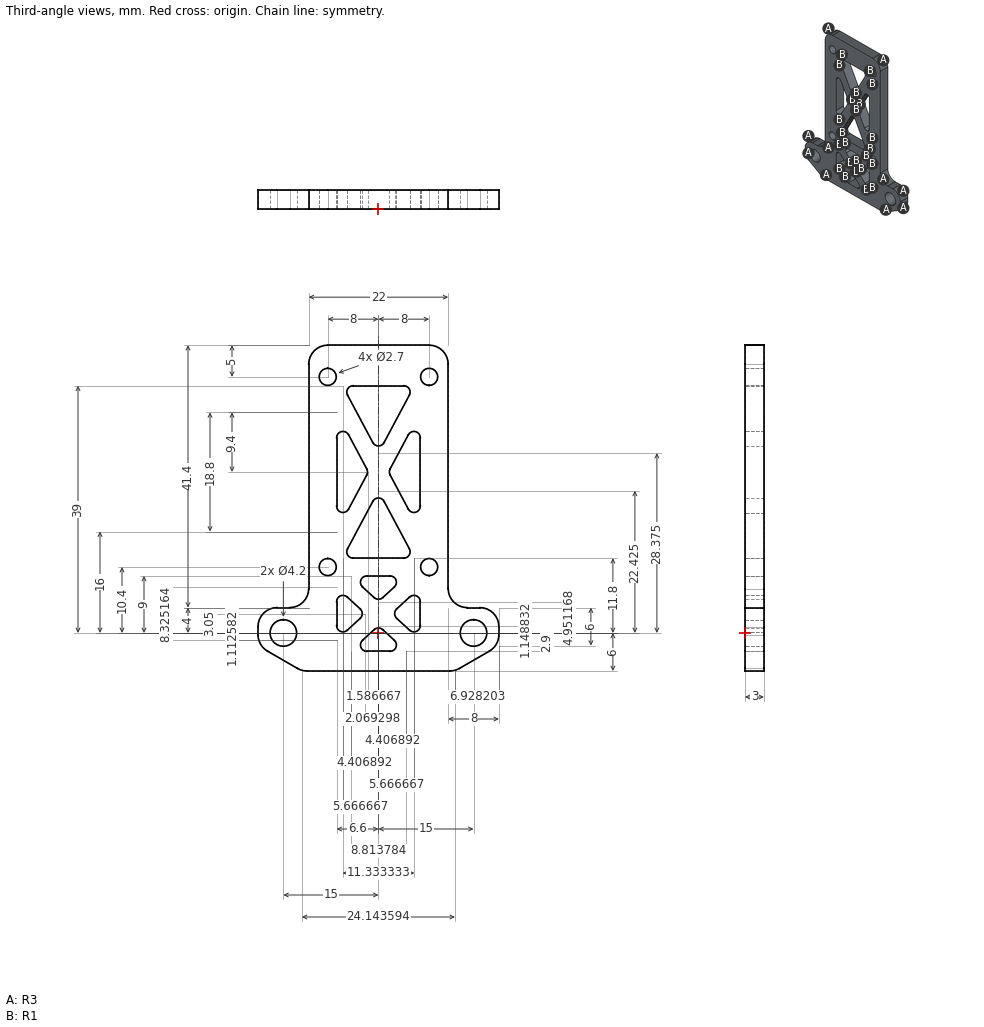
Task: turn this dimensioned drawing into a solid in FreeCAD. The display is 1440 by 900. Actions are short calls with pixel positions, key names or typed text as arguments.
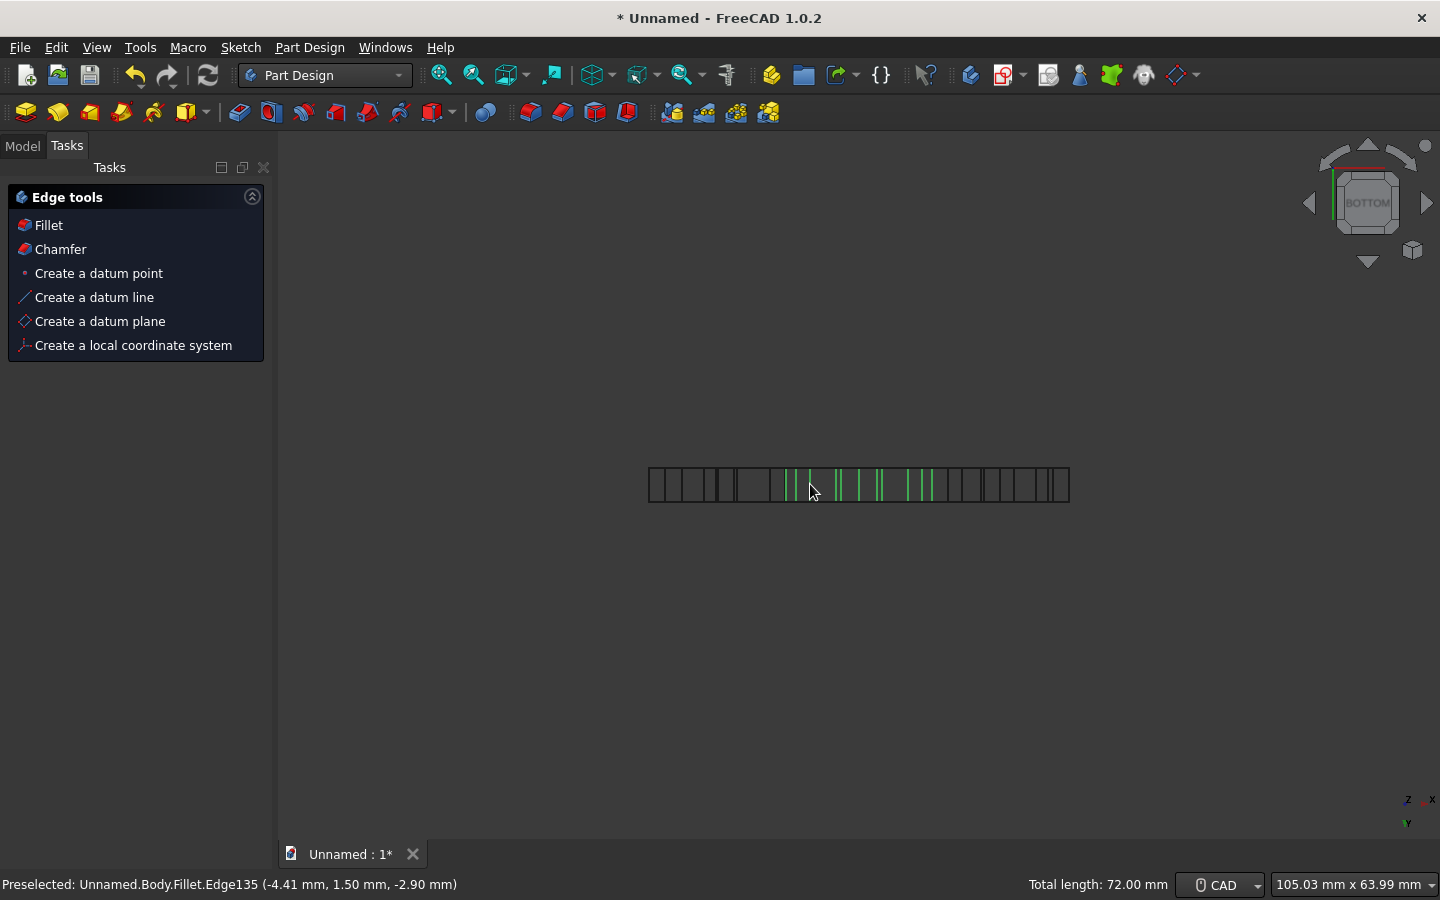
key(v)
key(1)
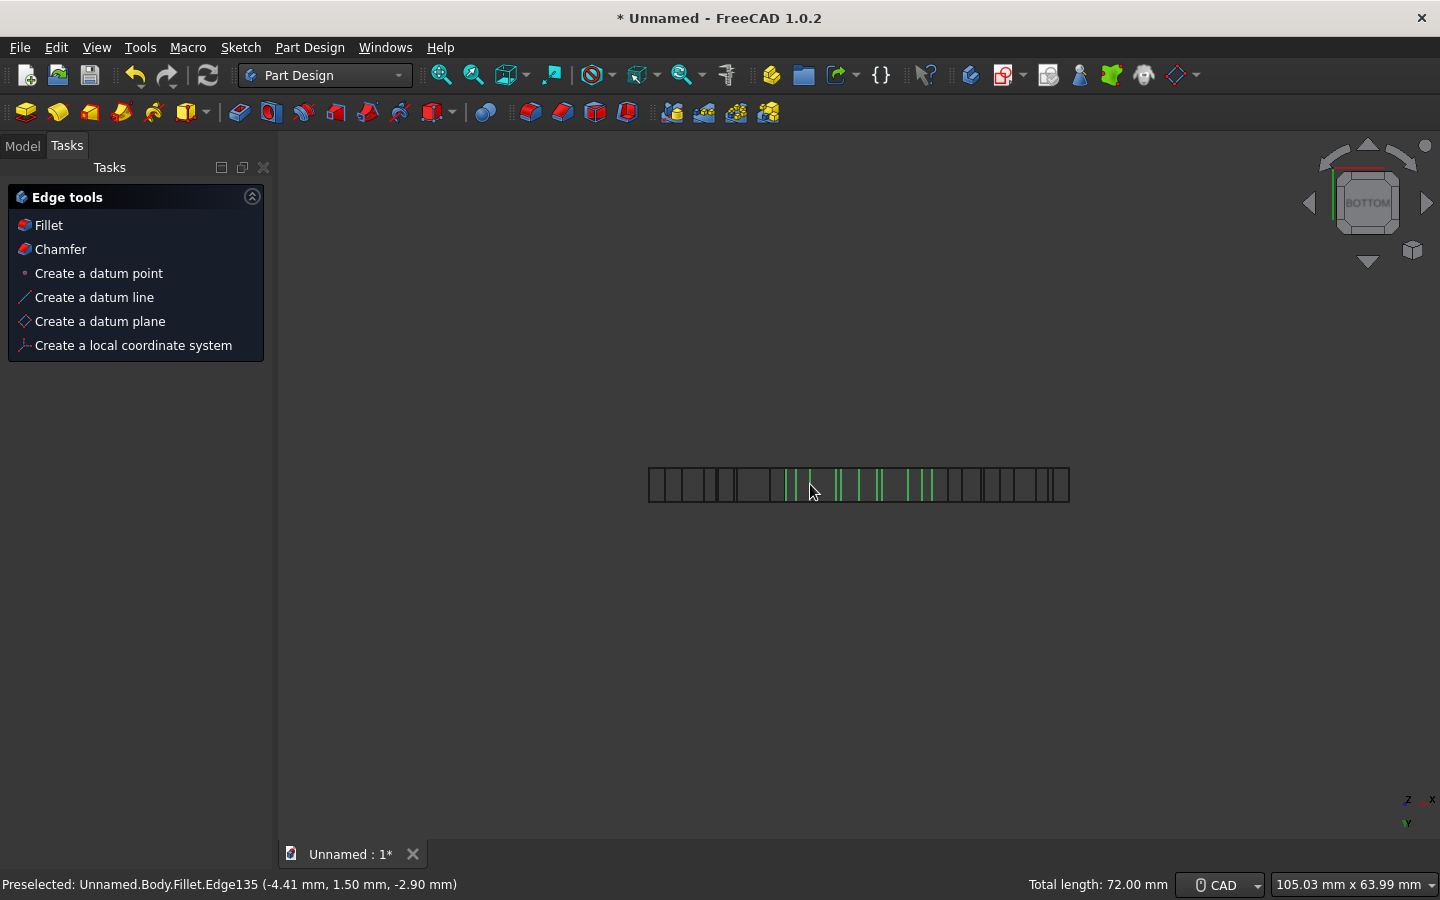
click(532, 112)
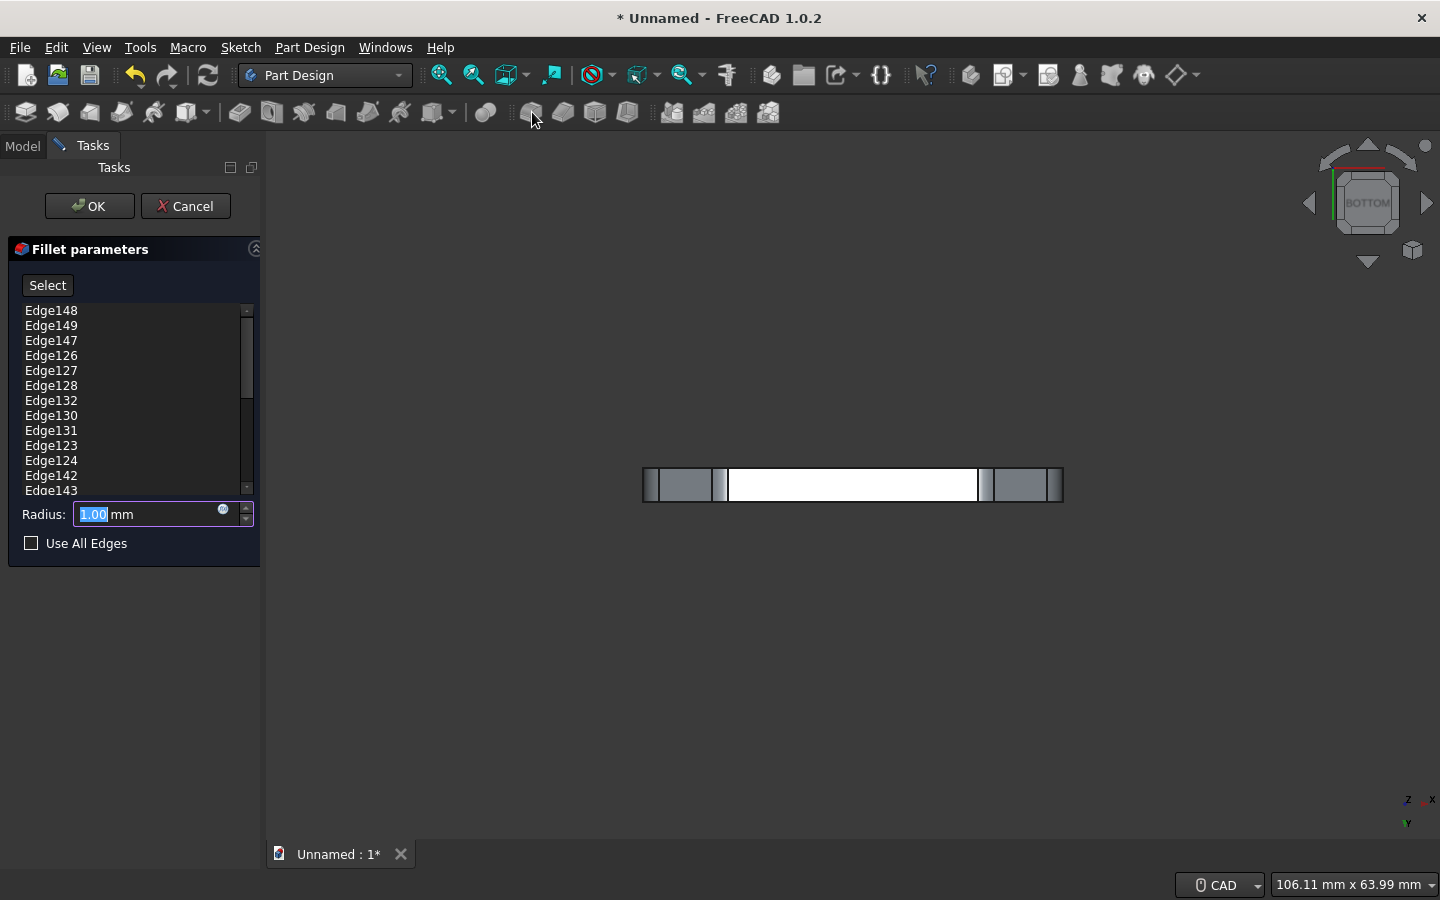
text(1)
key(Tab)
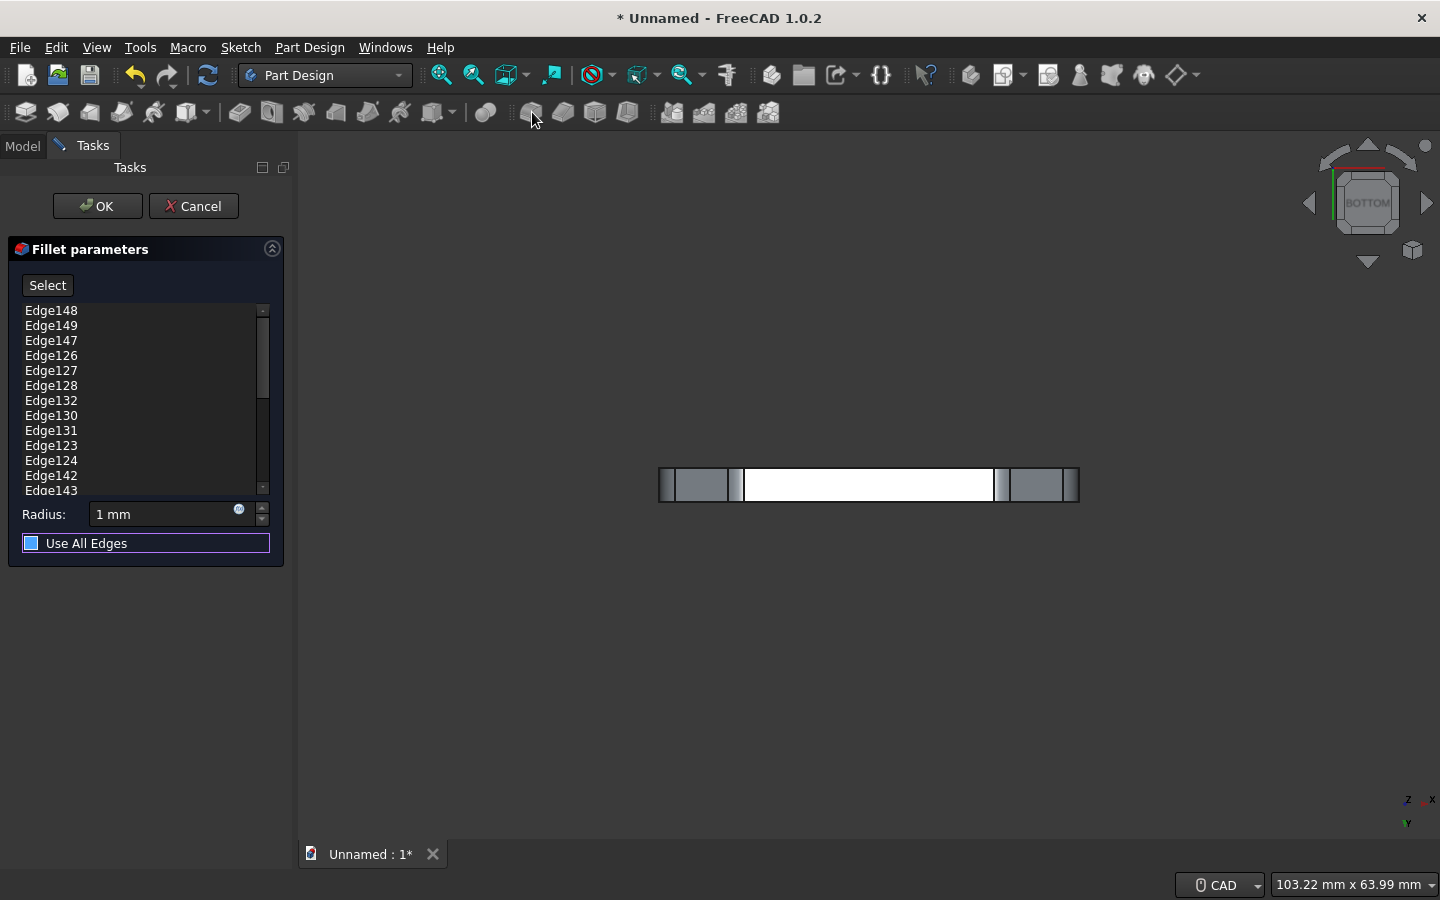
click(98, 206)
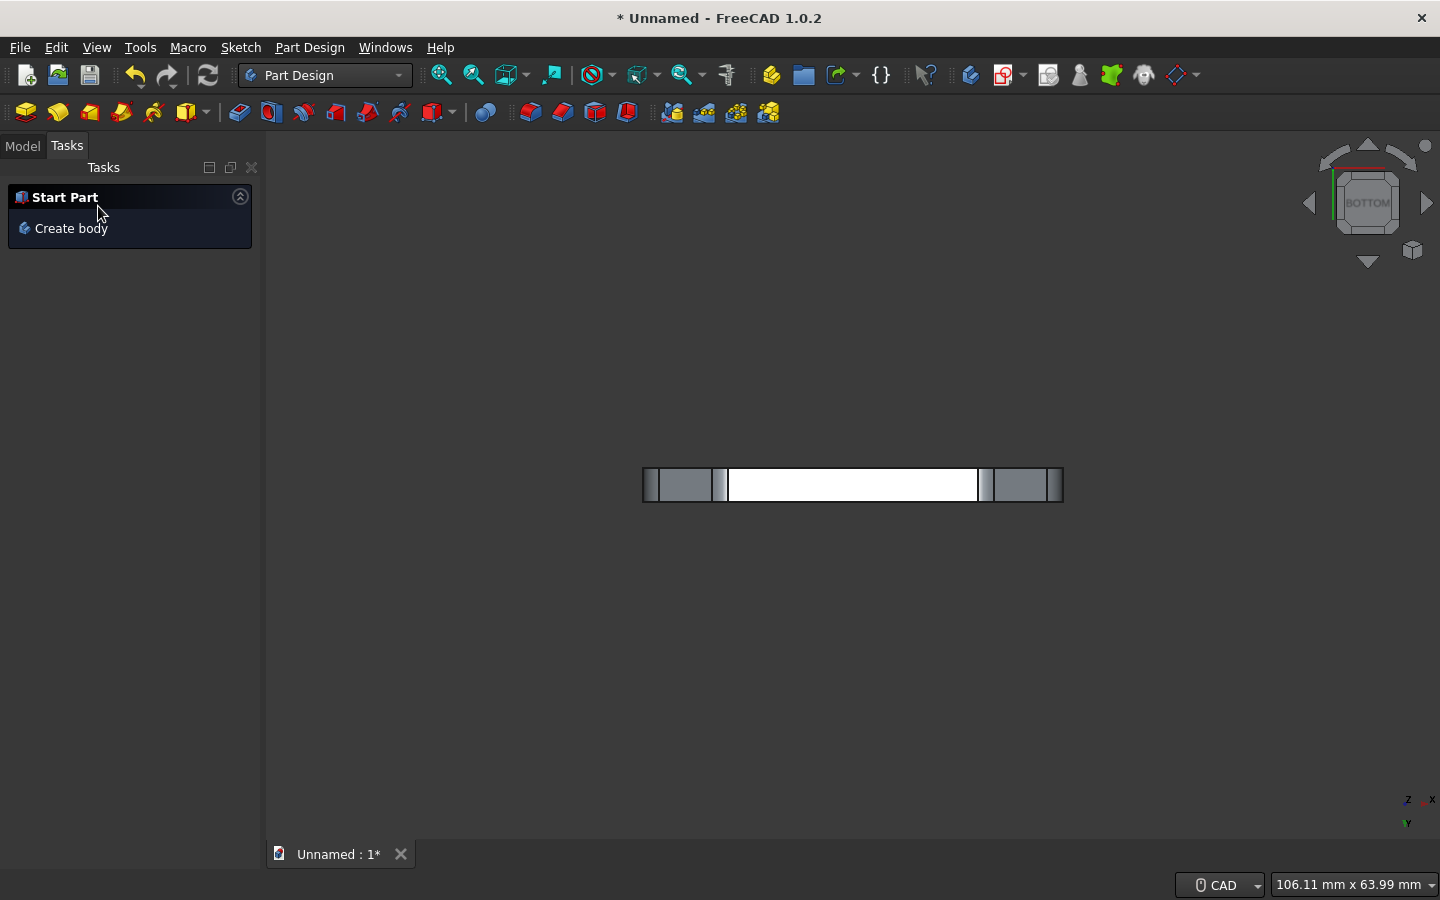
key(0)